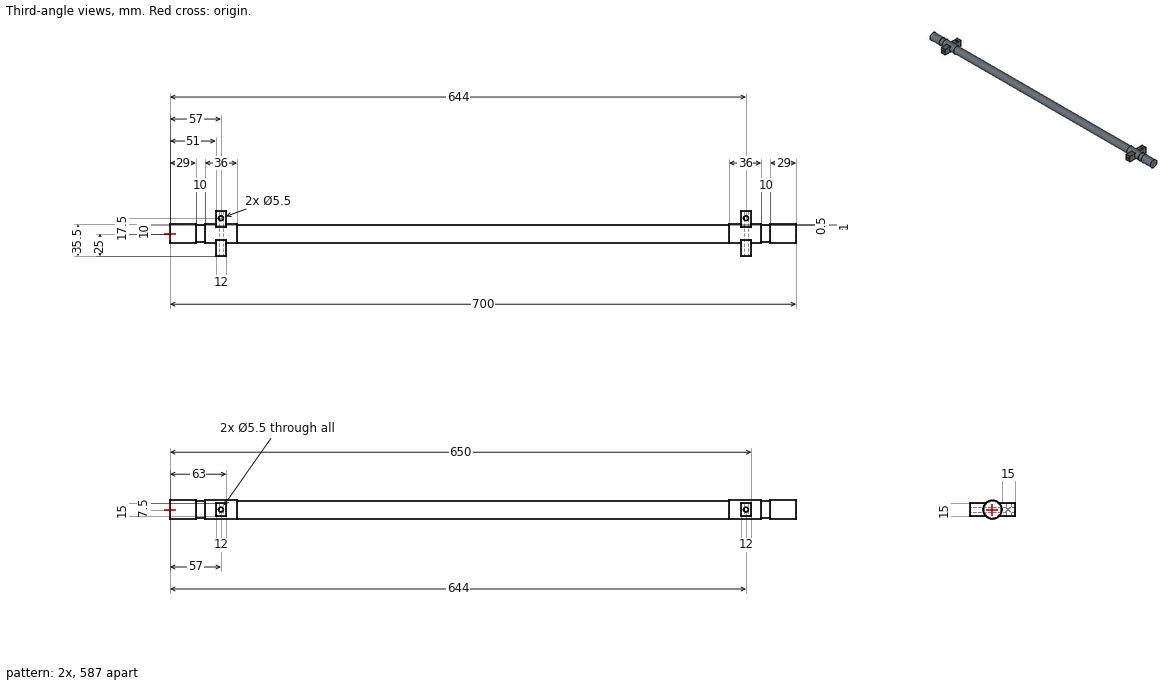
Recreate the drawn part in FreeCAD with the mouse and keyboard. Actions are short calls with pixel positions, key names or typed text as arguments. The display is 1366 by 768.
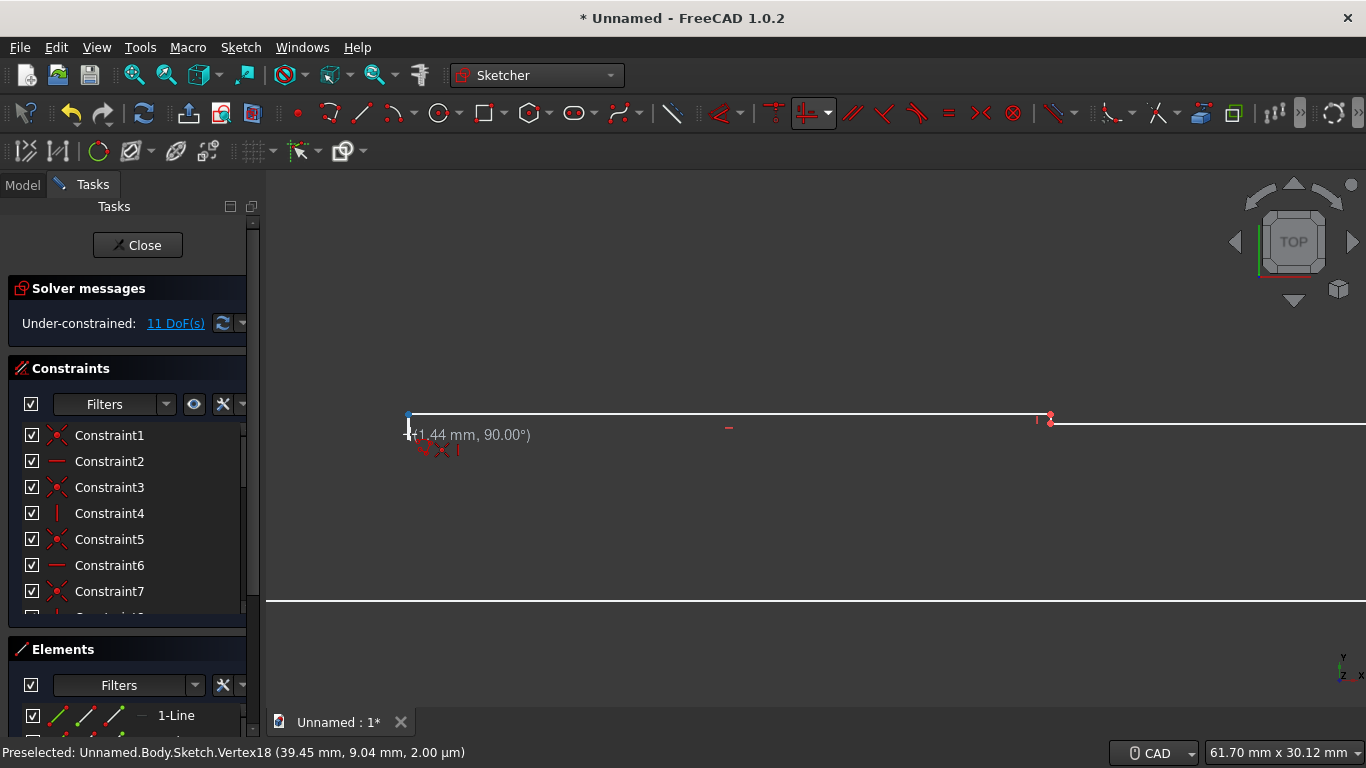
click(409, 432)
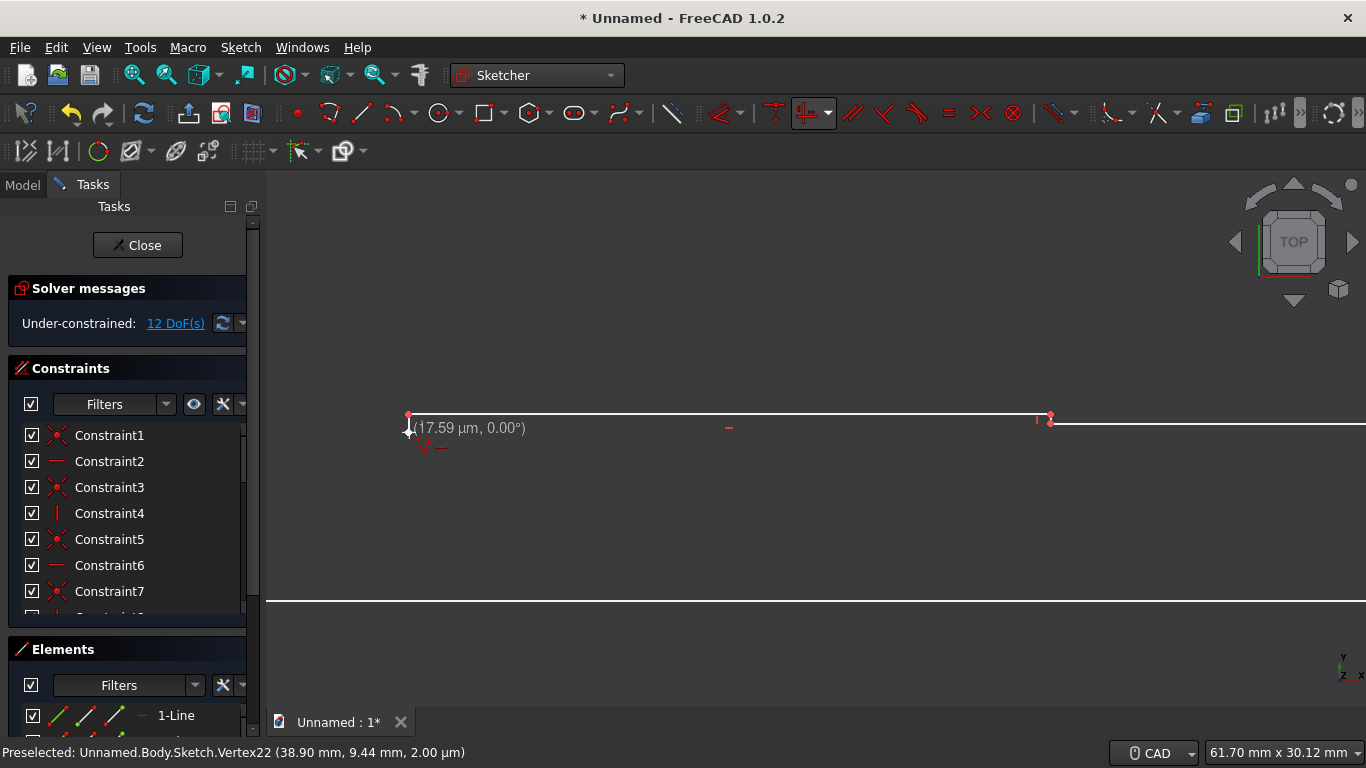
scroll(475, 435, down, 15)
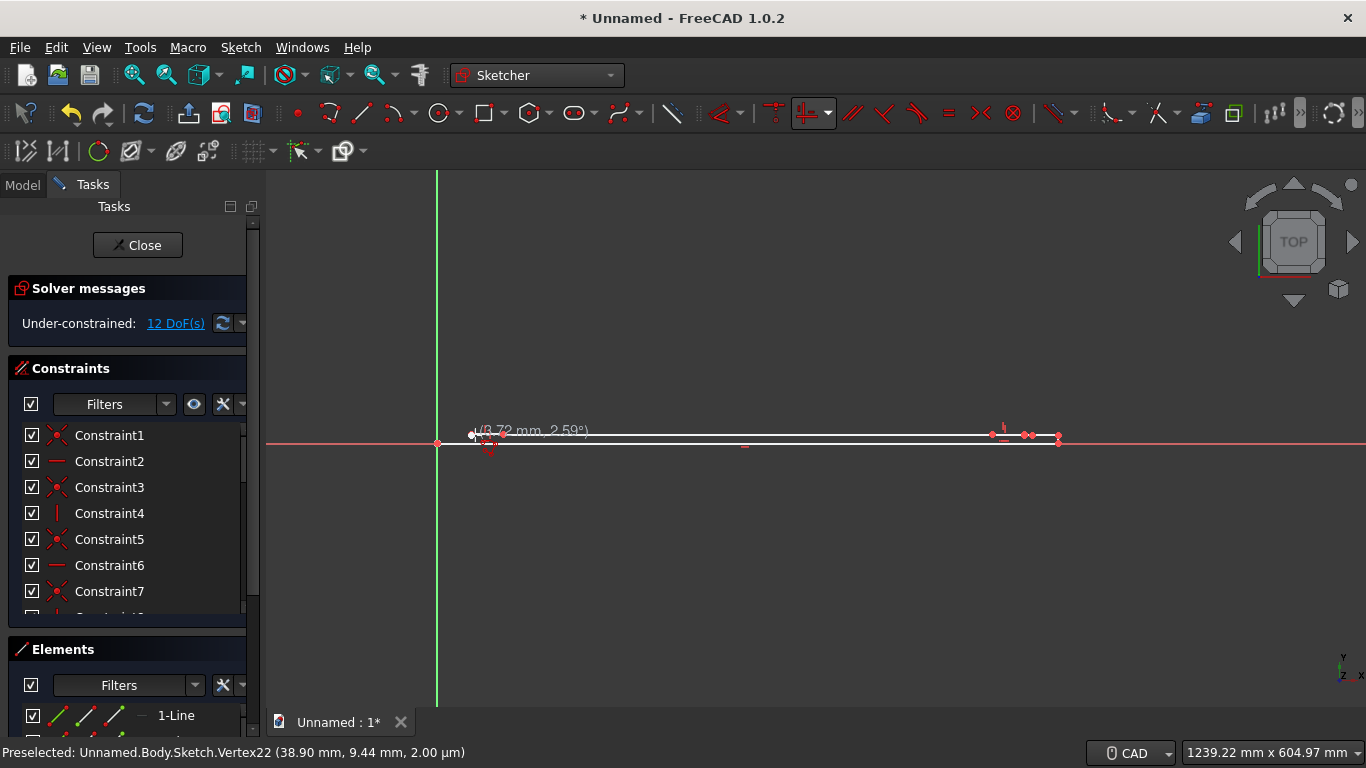
scroll(463, 435, up, 4)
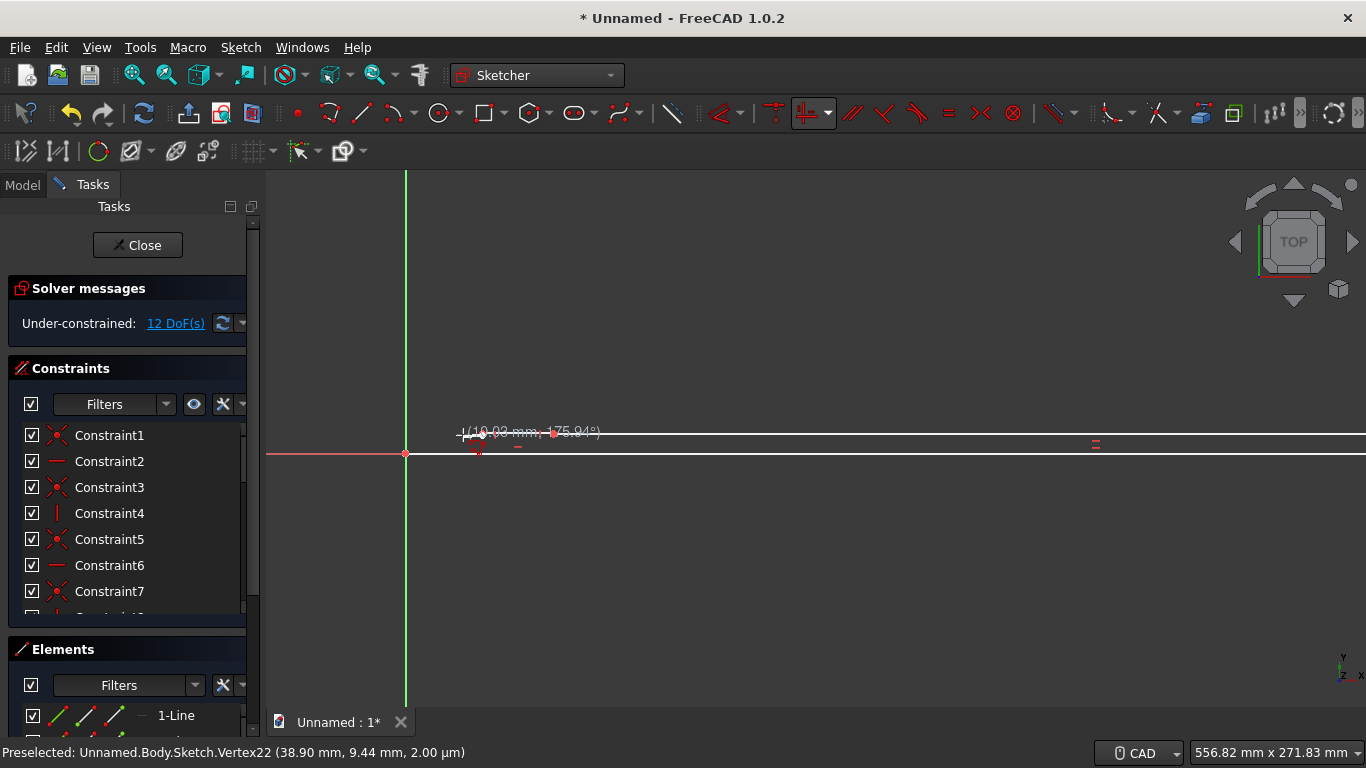
click(463, 435)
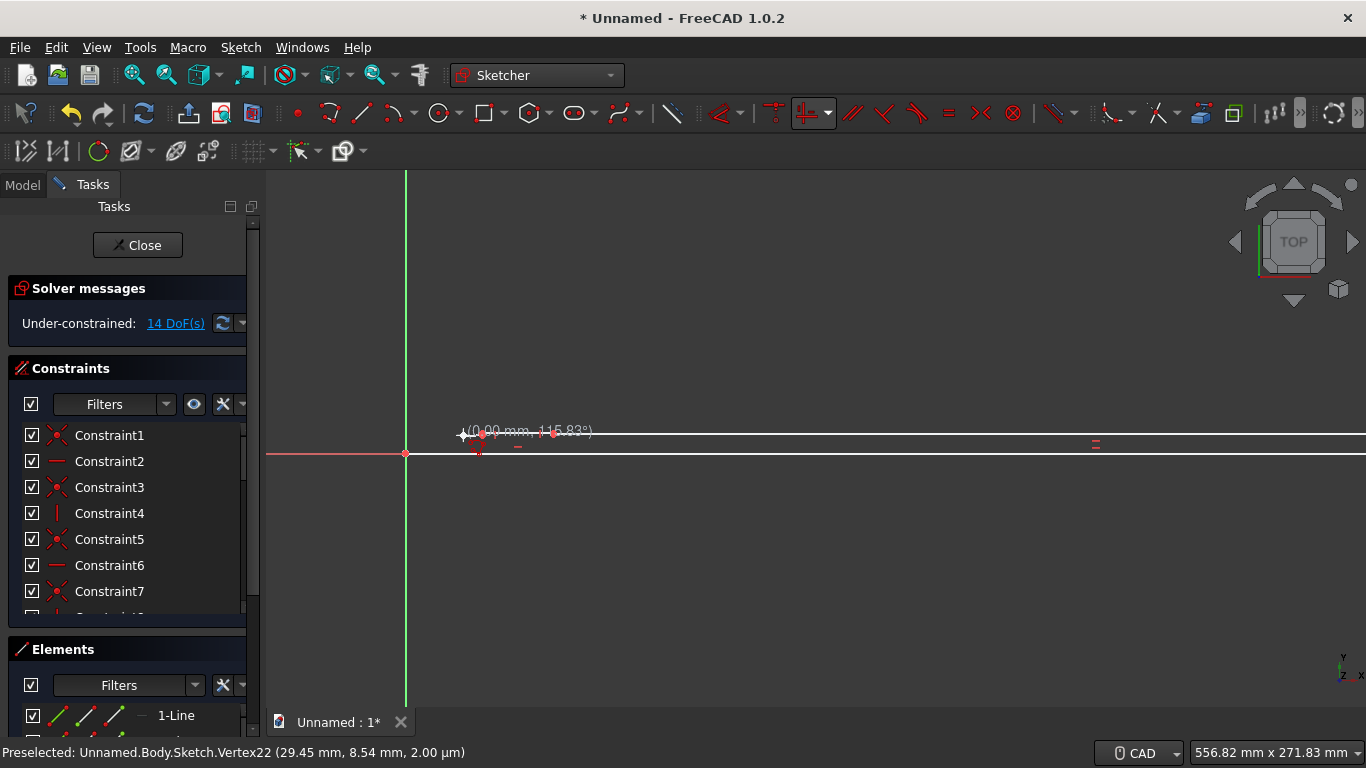
scroll(463, 433, up, 11)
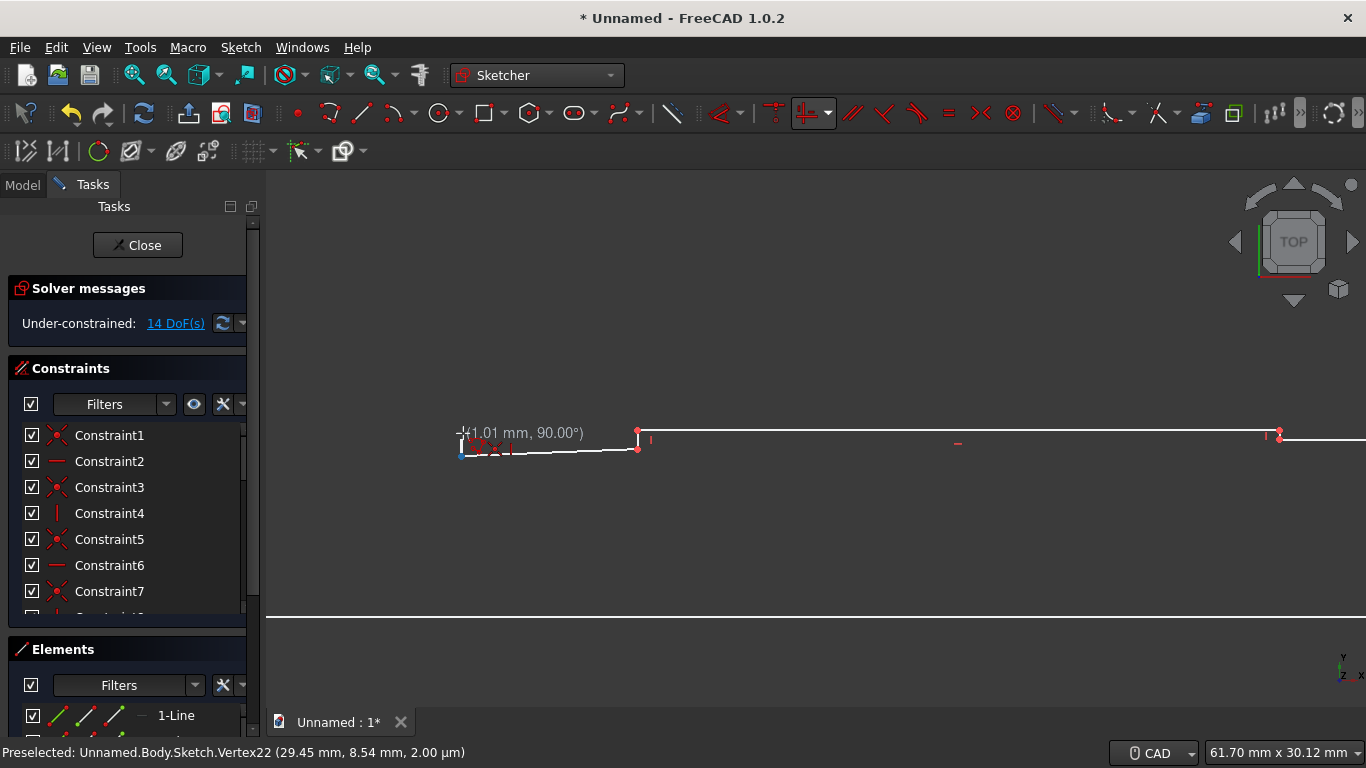
click(462, 430)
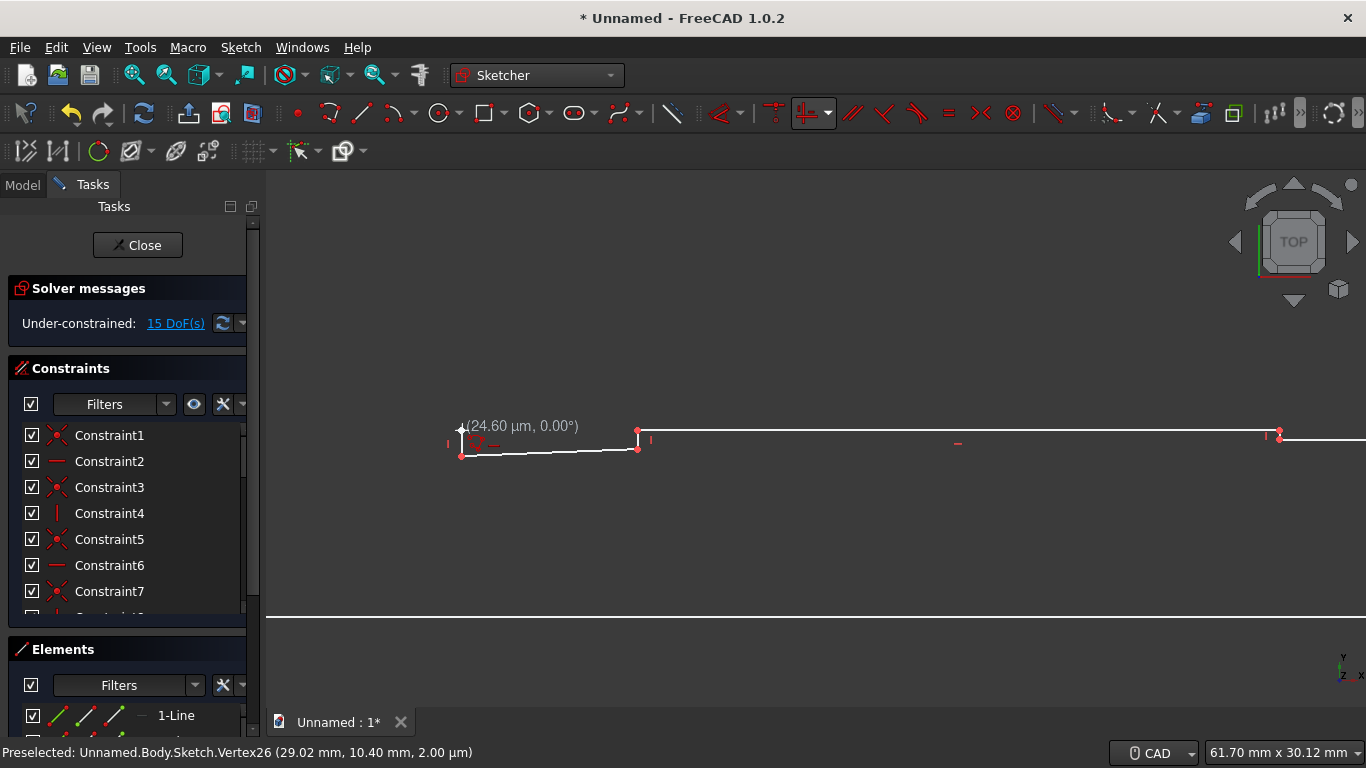
scroll(463, 434, down, 15)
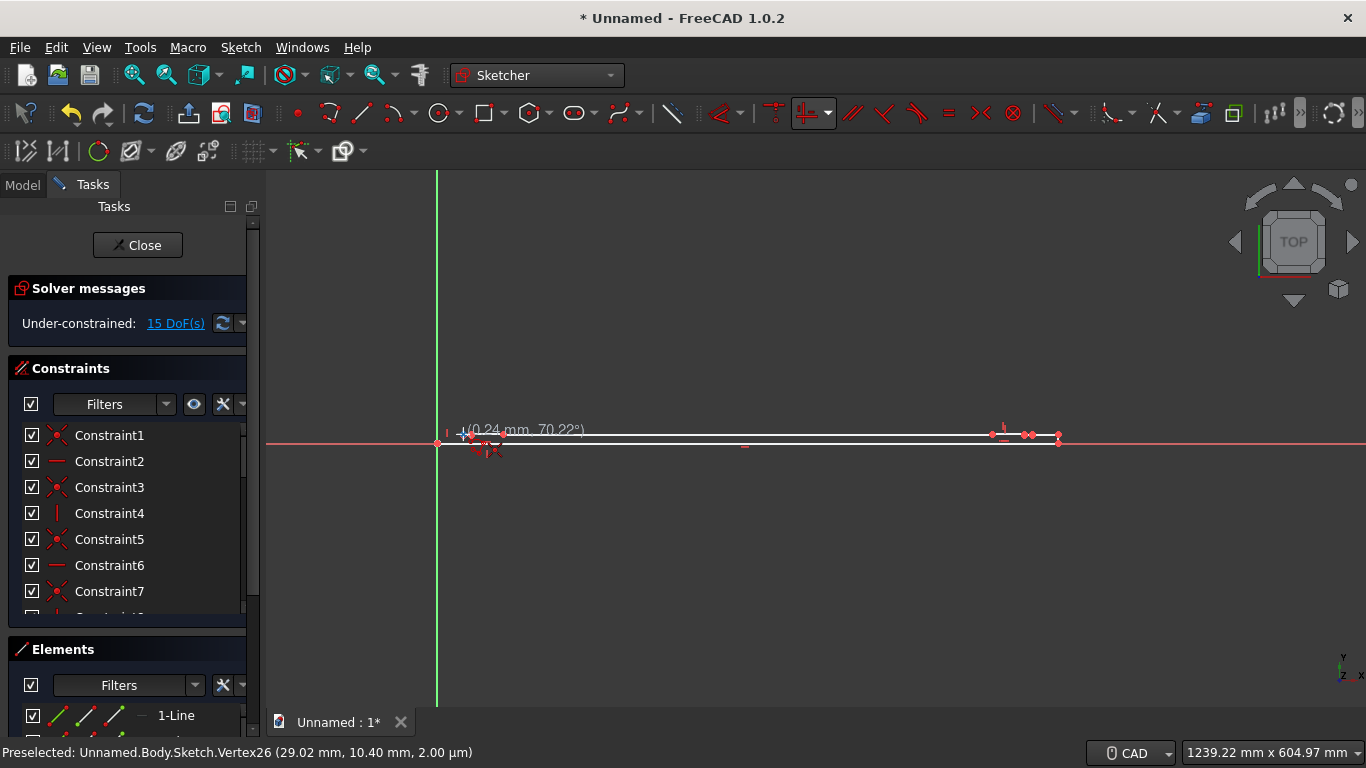
scroll(437, 434, up, 3)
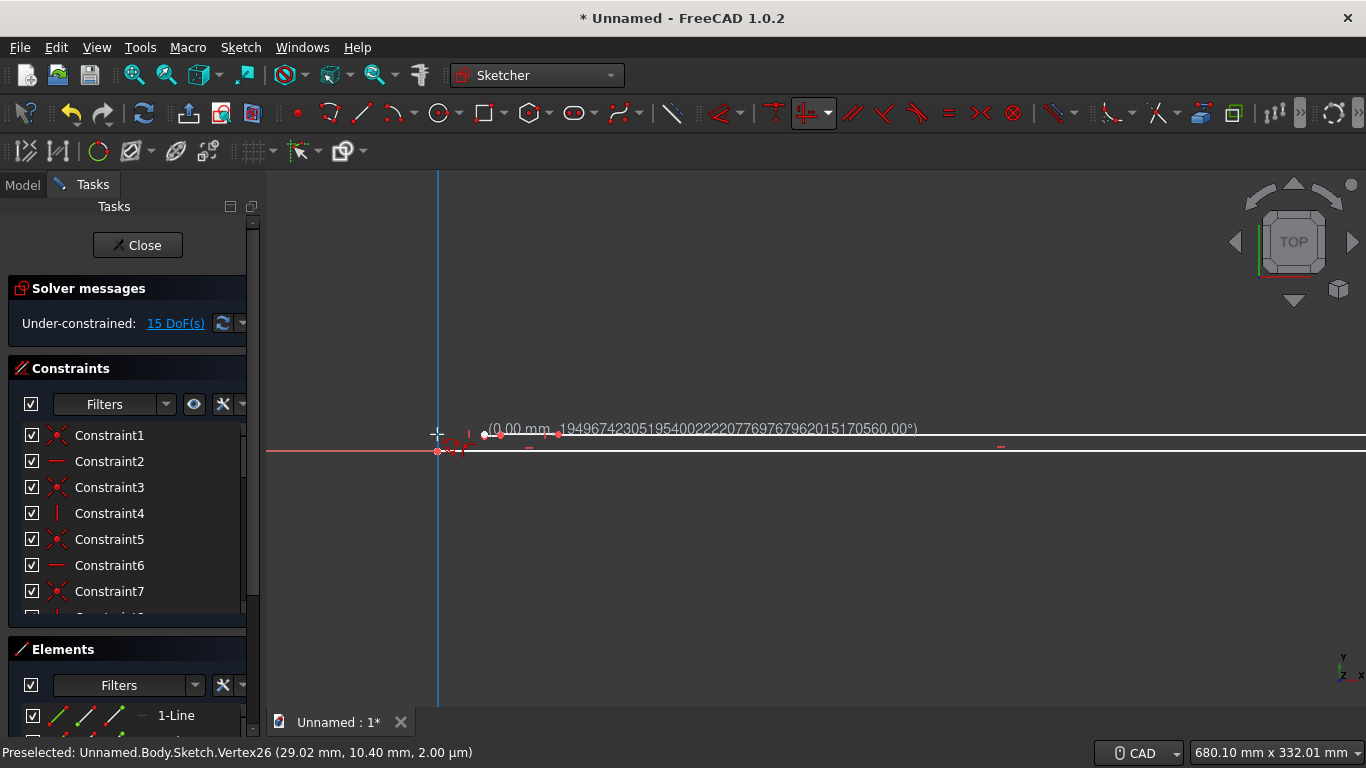
click(447, 434)
click(438, 451)
key(Escape)
key(Escape)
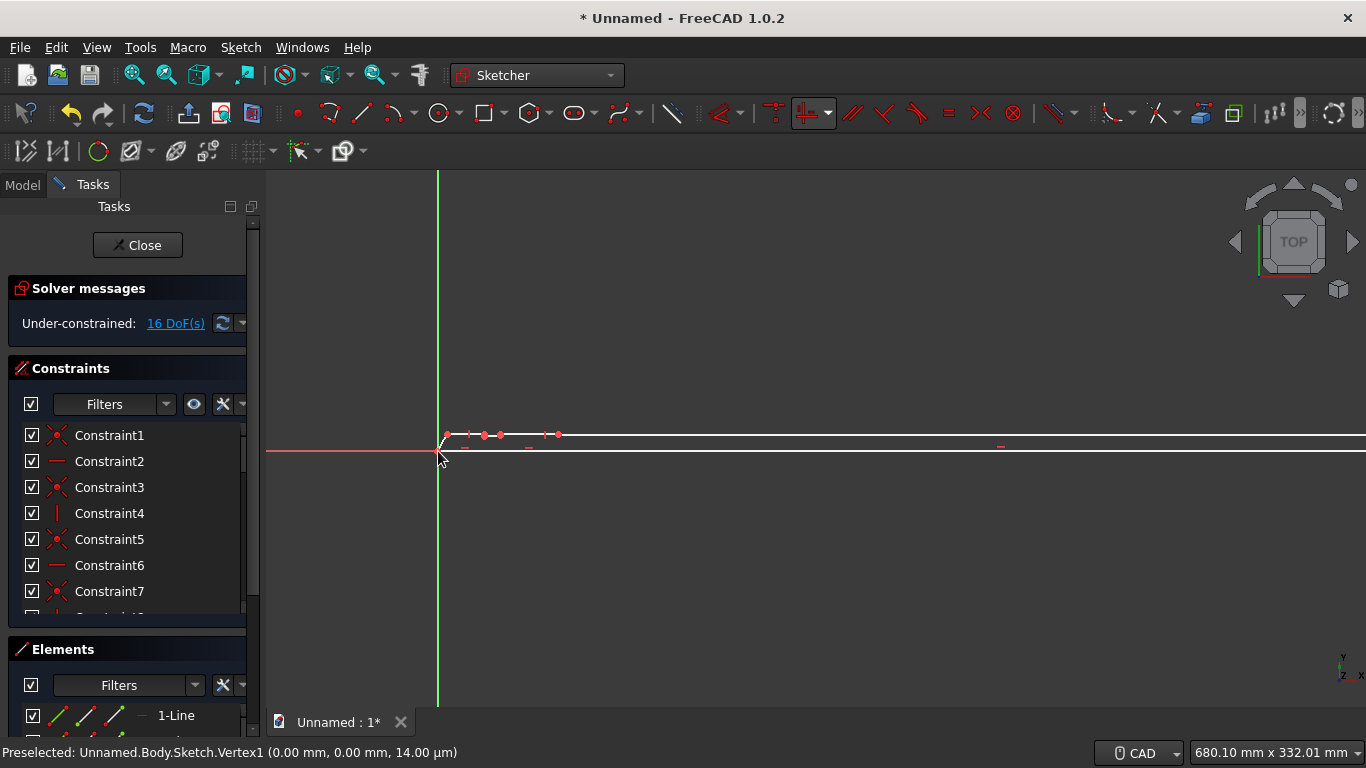
scroll(492, 436, up, 3)